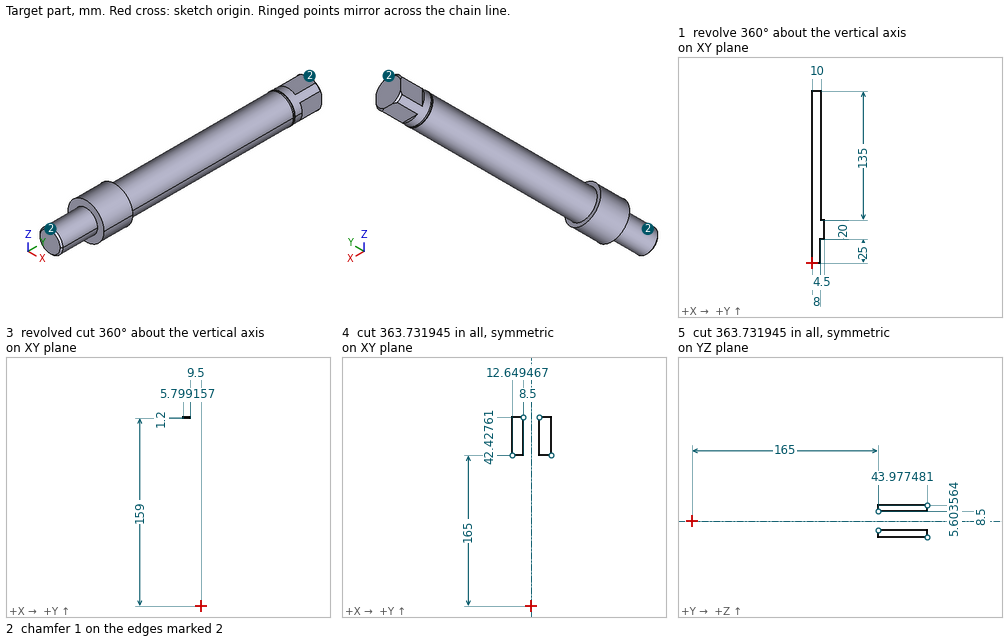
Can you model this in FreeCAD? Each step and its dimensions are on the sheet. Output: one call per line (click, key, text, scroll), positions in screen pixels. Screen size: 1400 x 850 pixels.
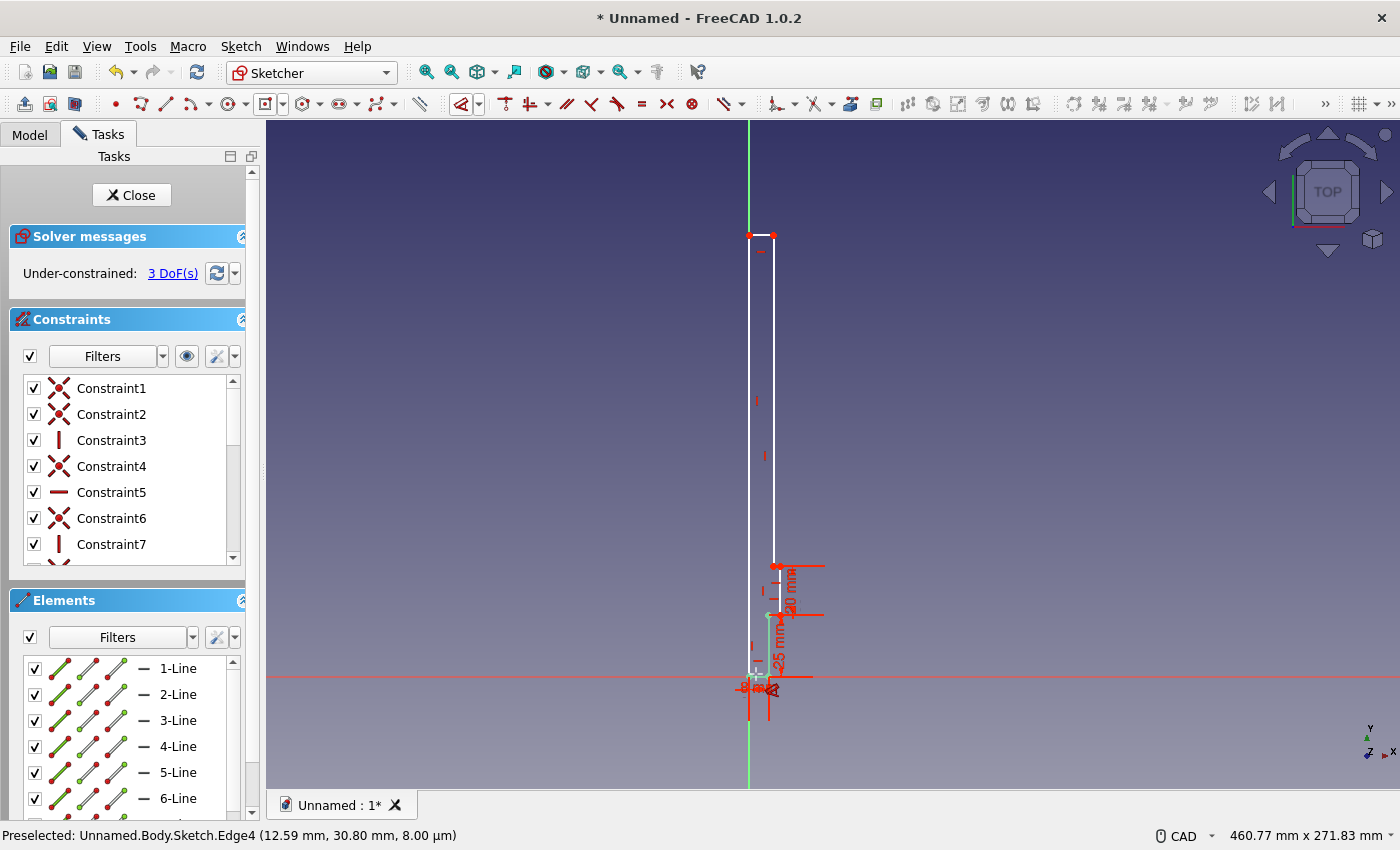
scroll(766, 235, up, 4)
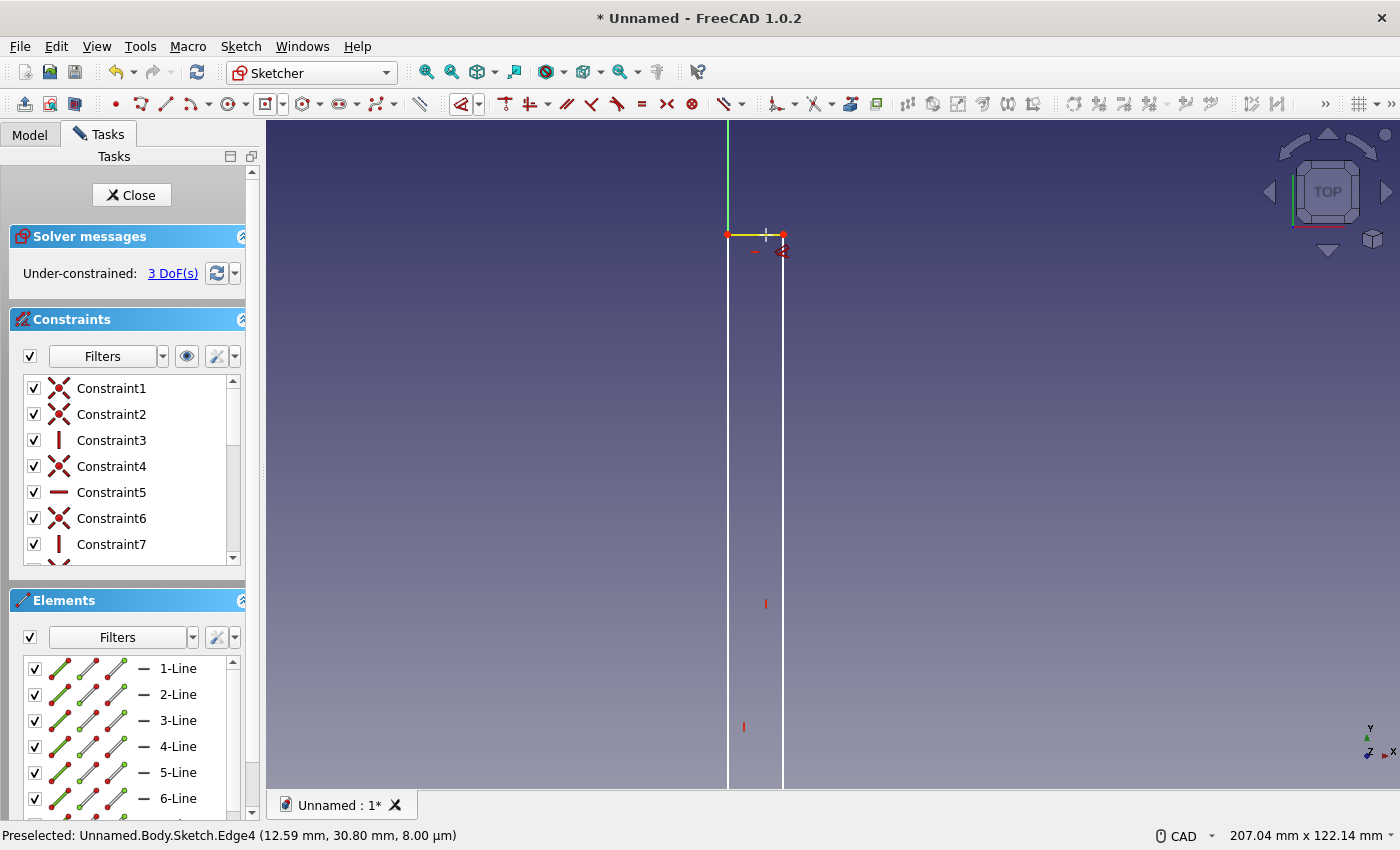
click(766, 235)
click(755, 201)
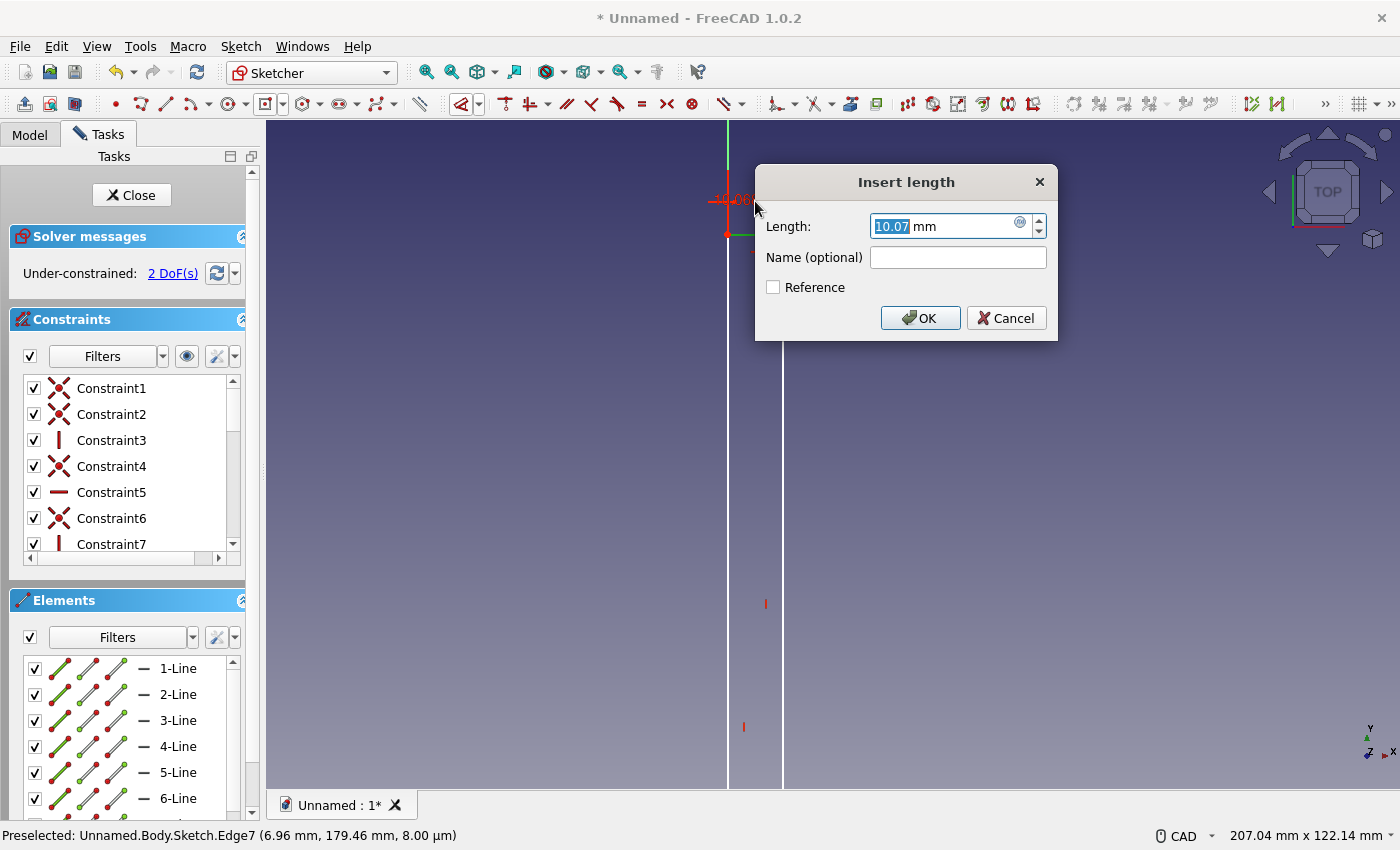
text(10)
key(Return)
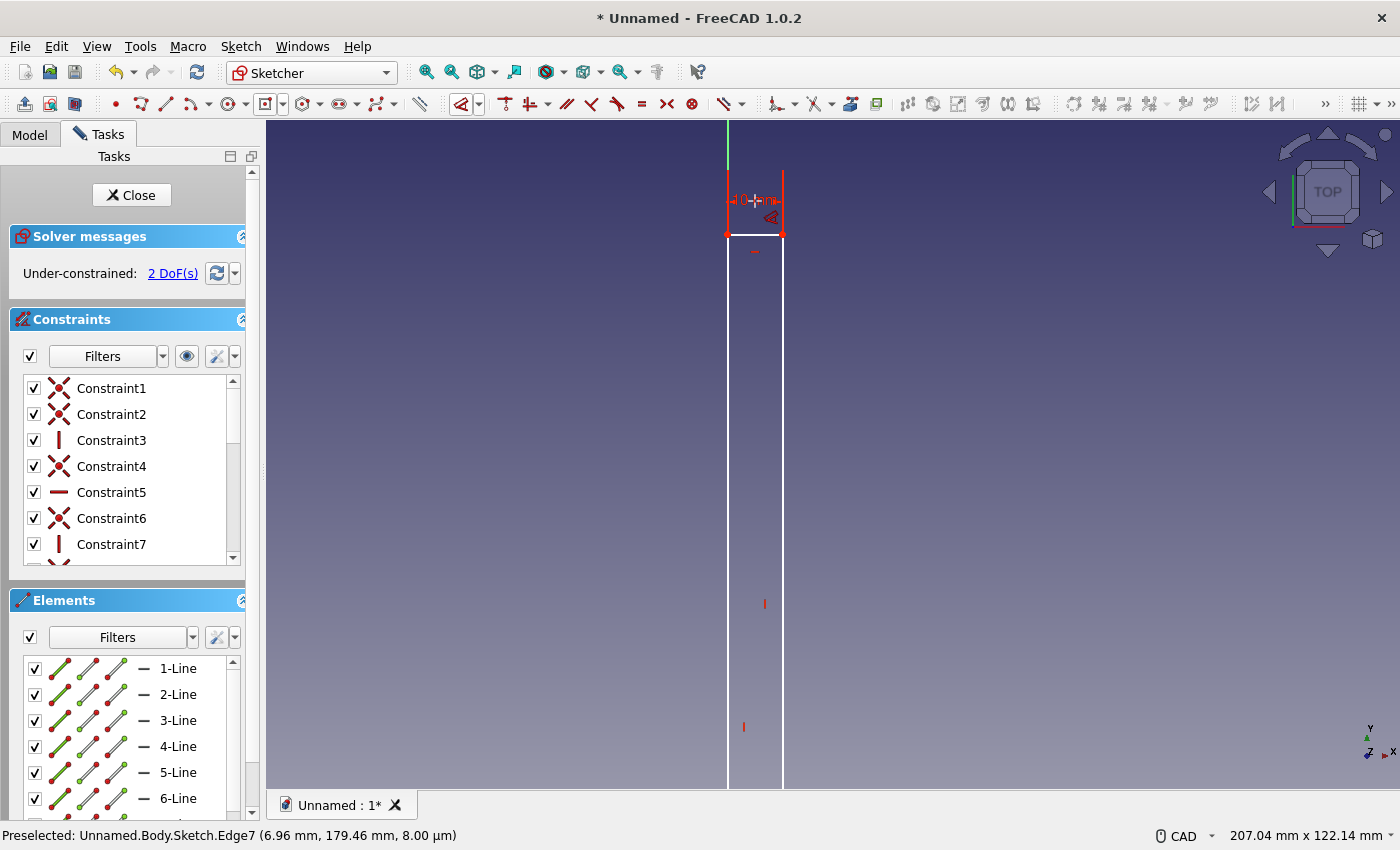
scroll(766, 234, down, 4)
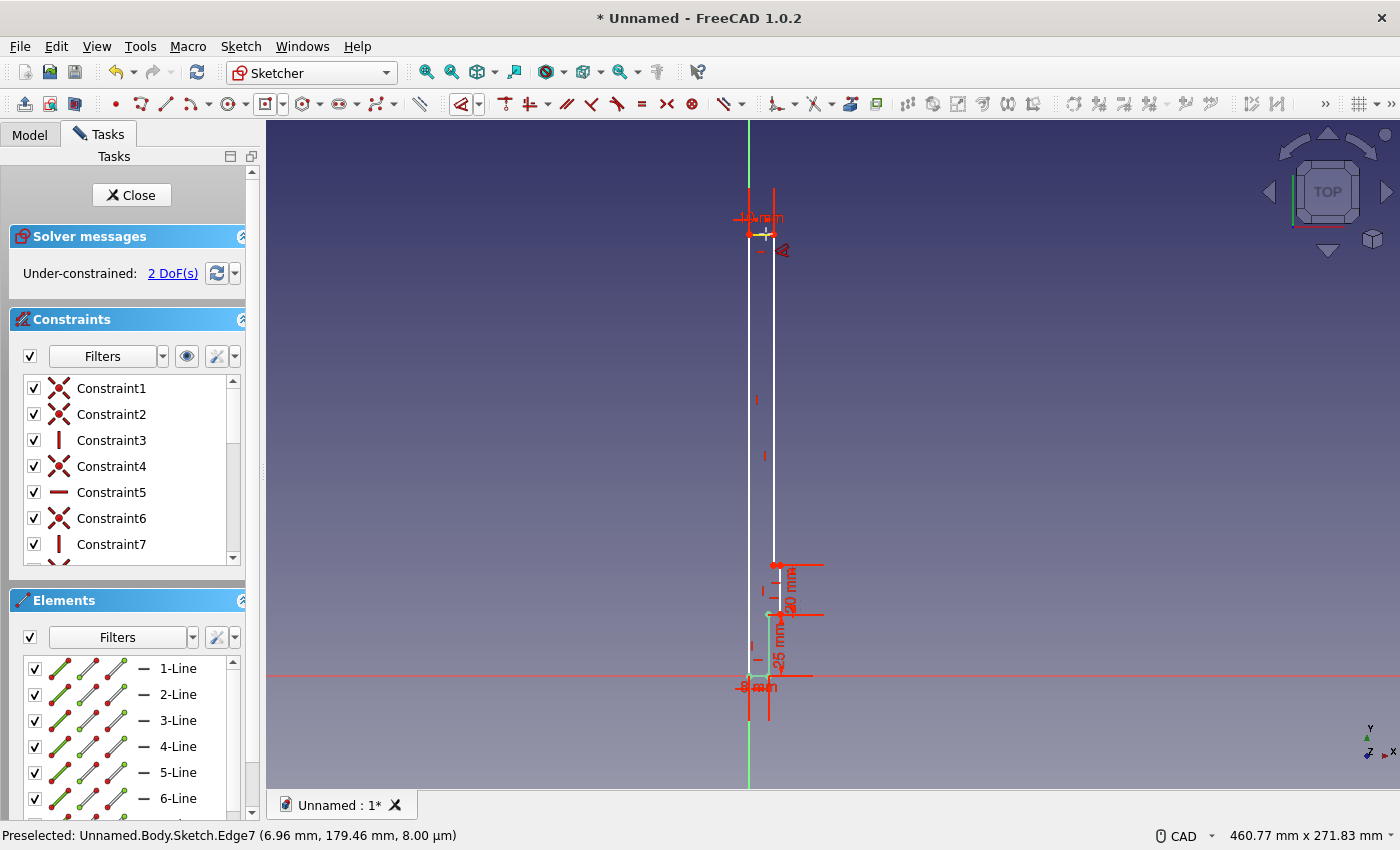
scroll(773, 615, up, 7)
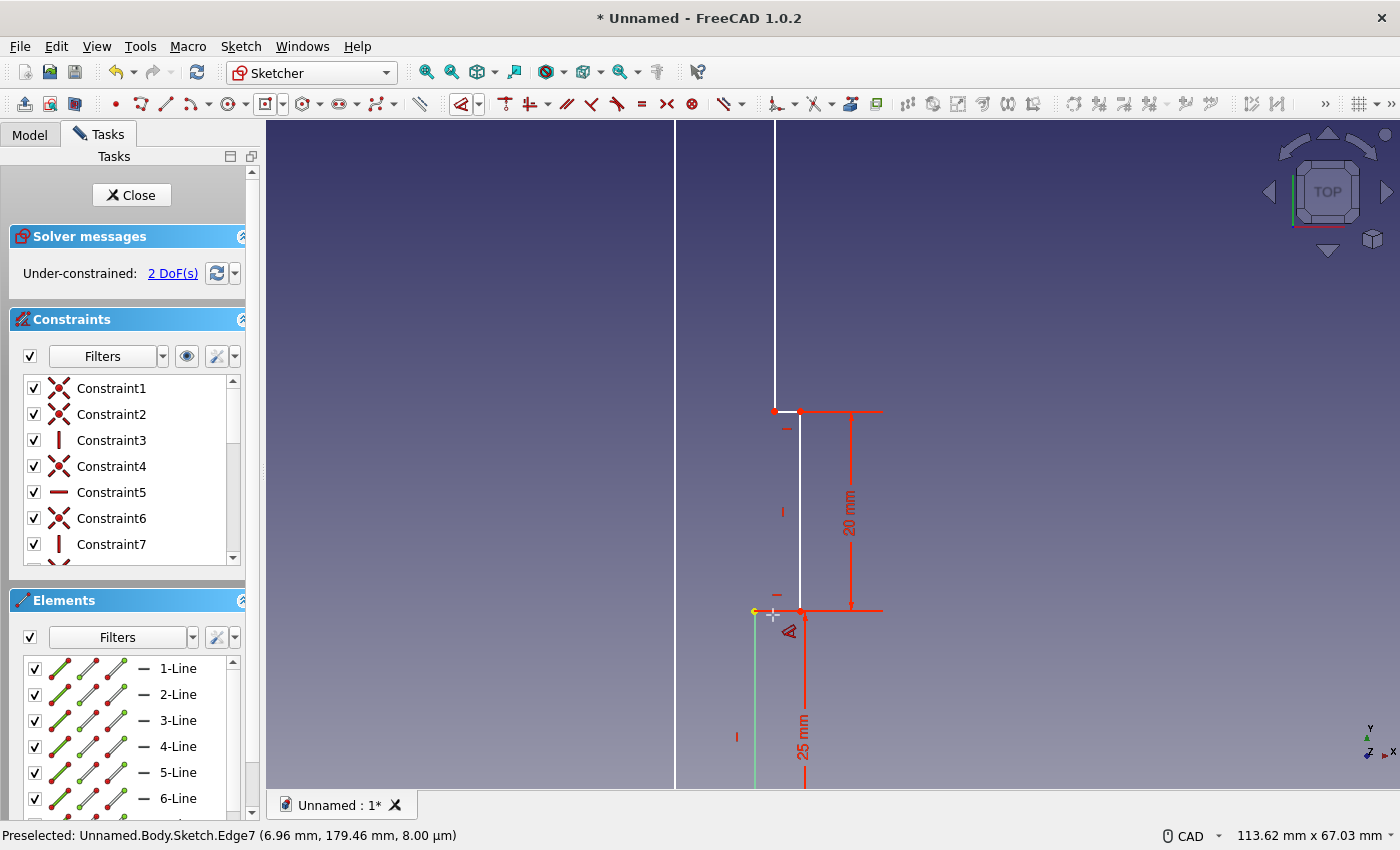
click(773, 611)
click(778, 645)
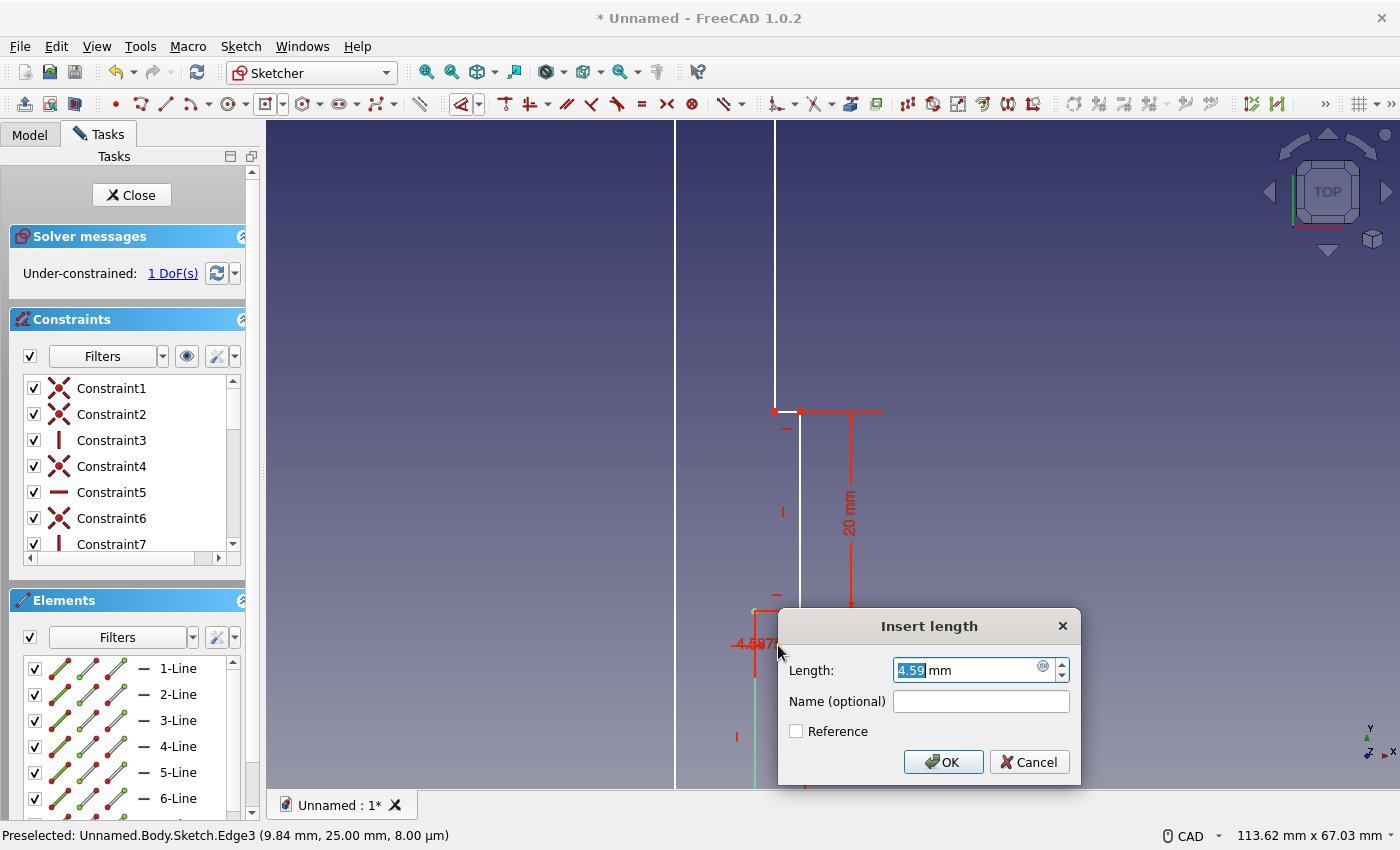
text(4.5)
key(Return)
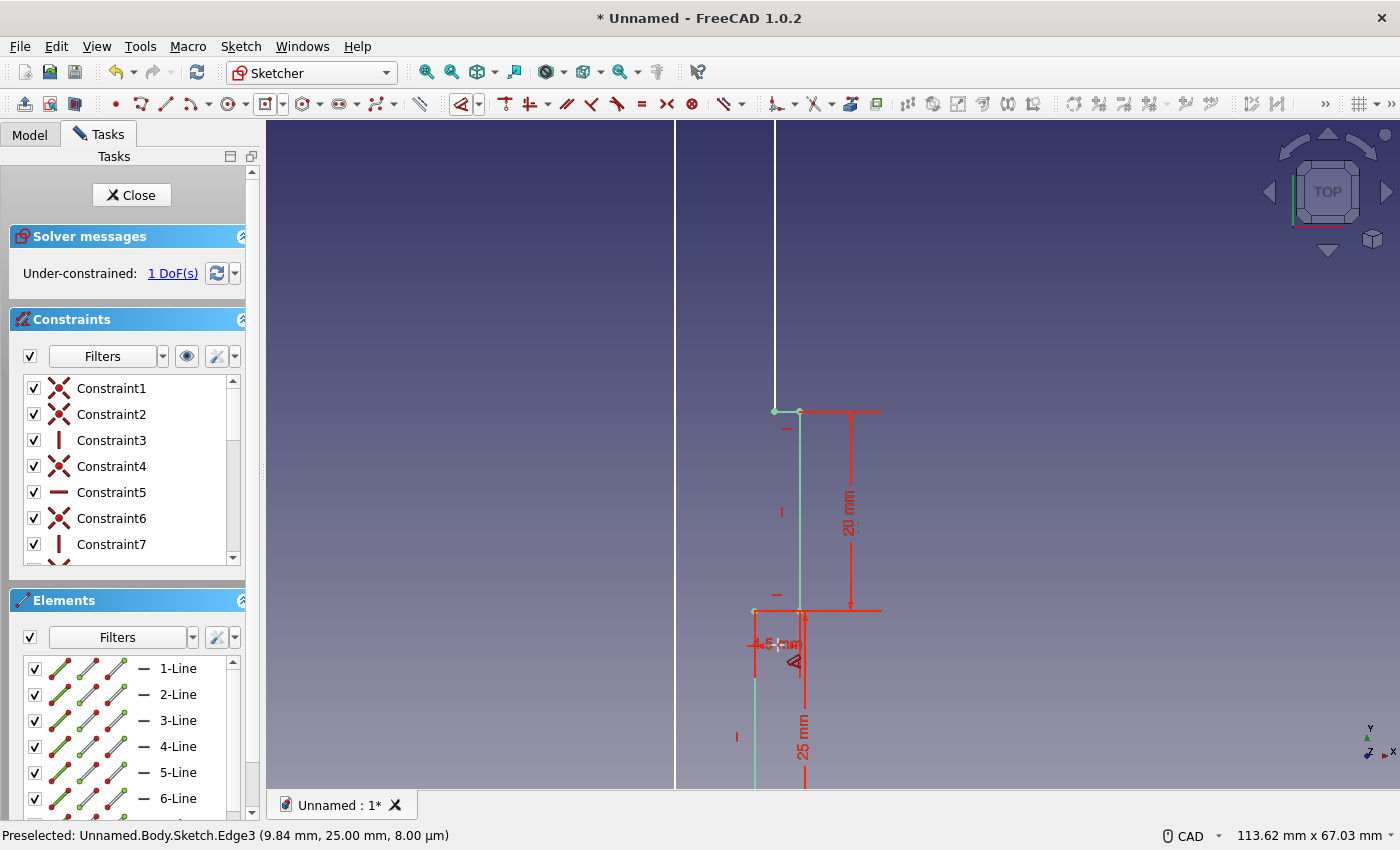
scroll(773, 615, down, 7)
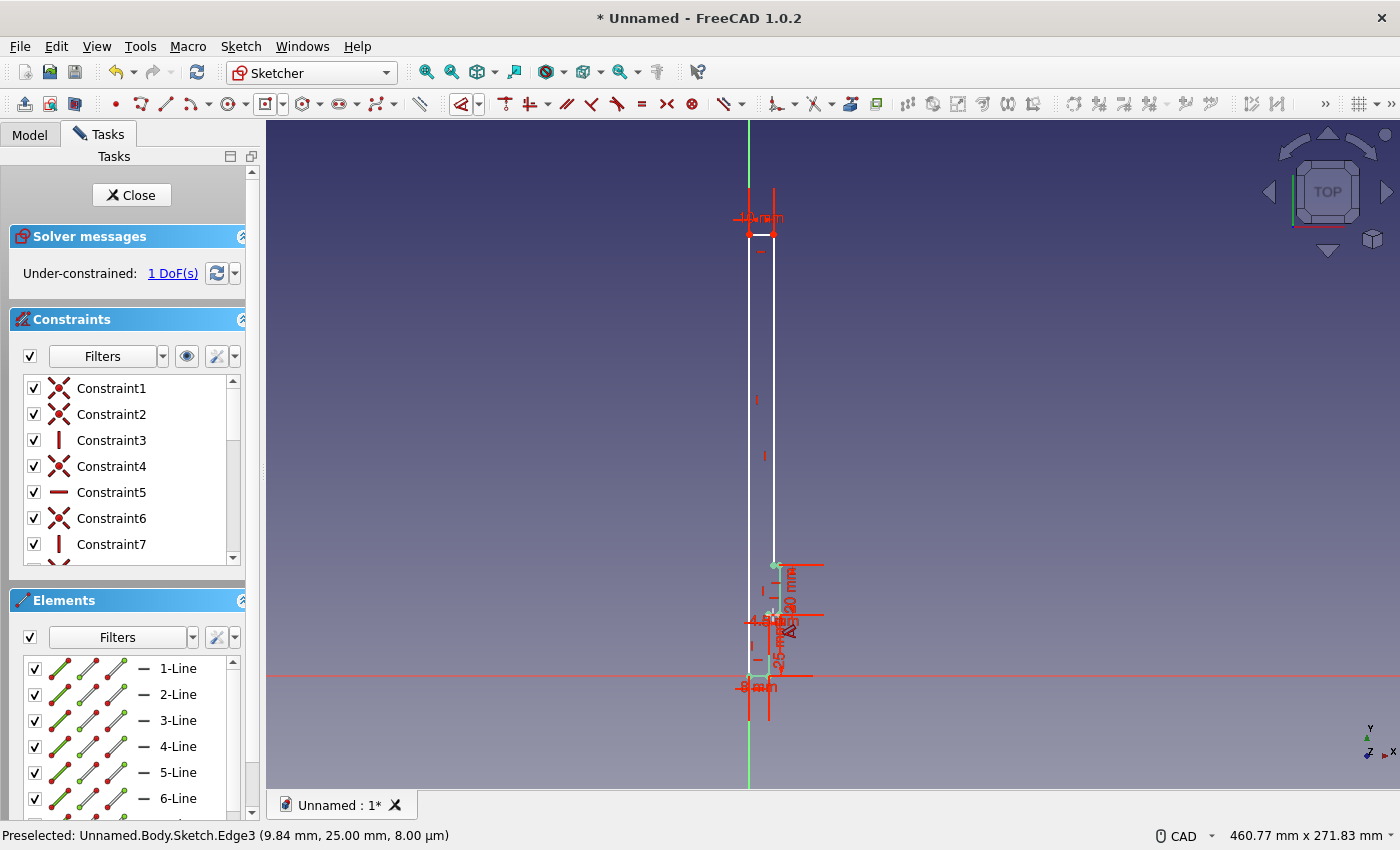
click(774, 466)
click(808, 400)